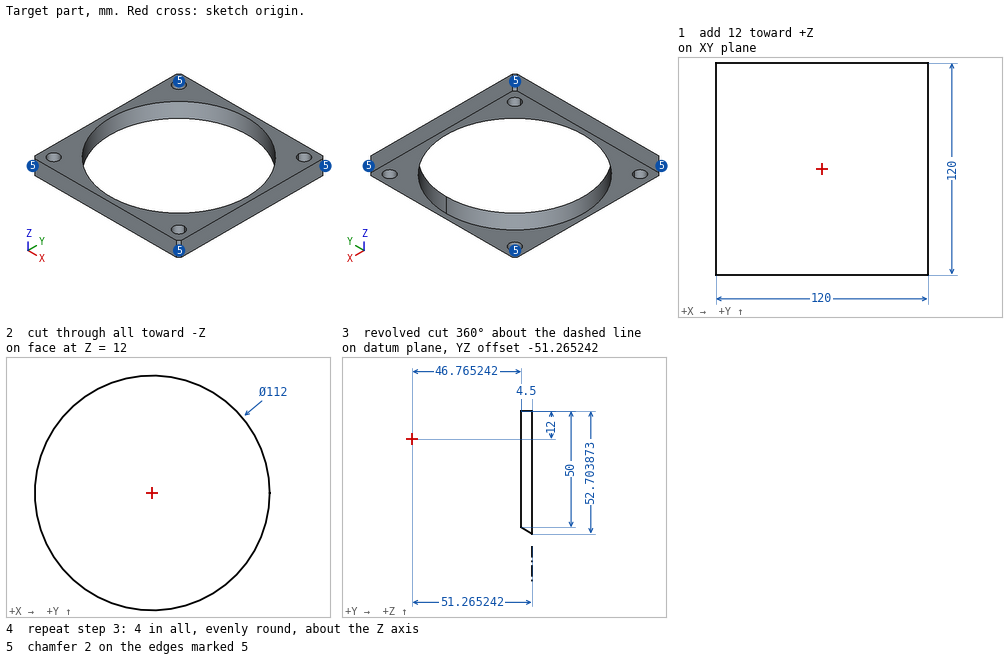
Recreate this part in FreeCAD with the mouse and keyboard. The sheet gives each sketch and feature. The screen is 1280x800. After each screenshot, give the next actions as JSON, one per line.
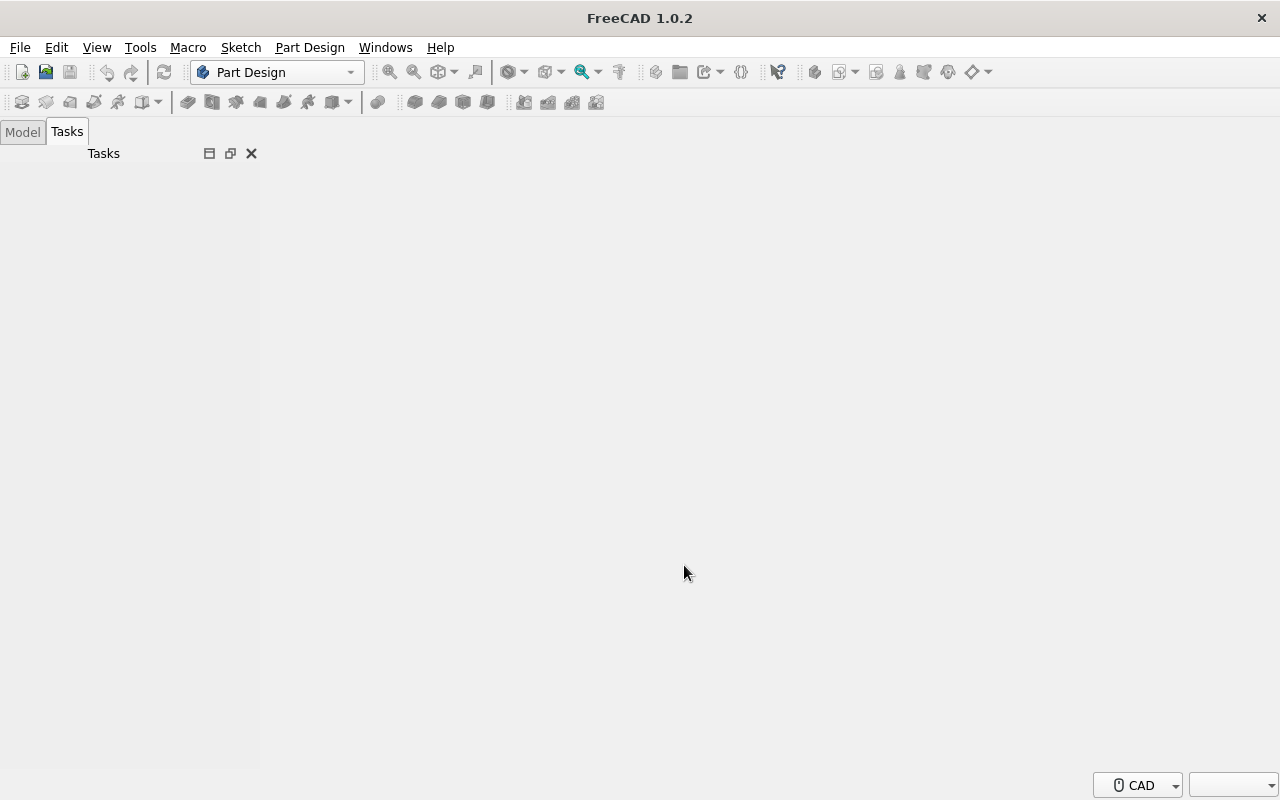
{"action": "key", "text": "ctrl+n"}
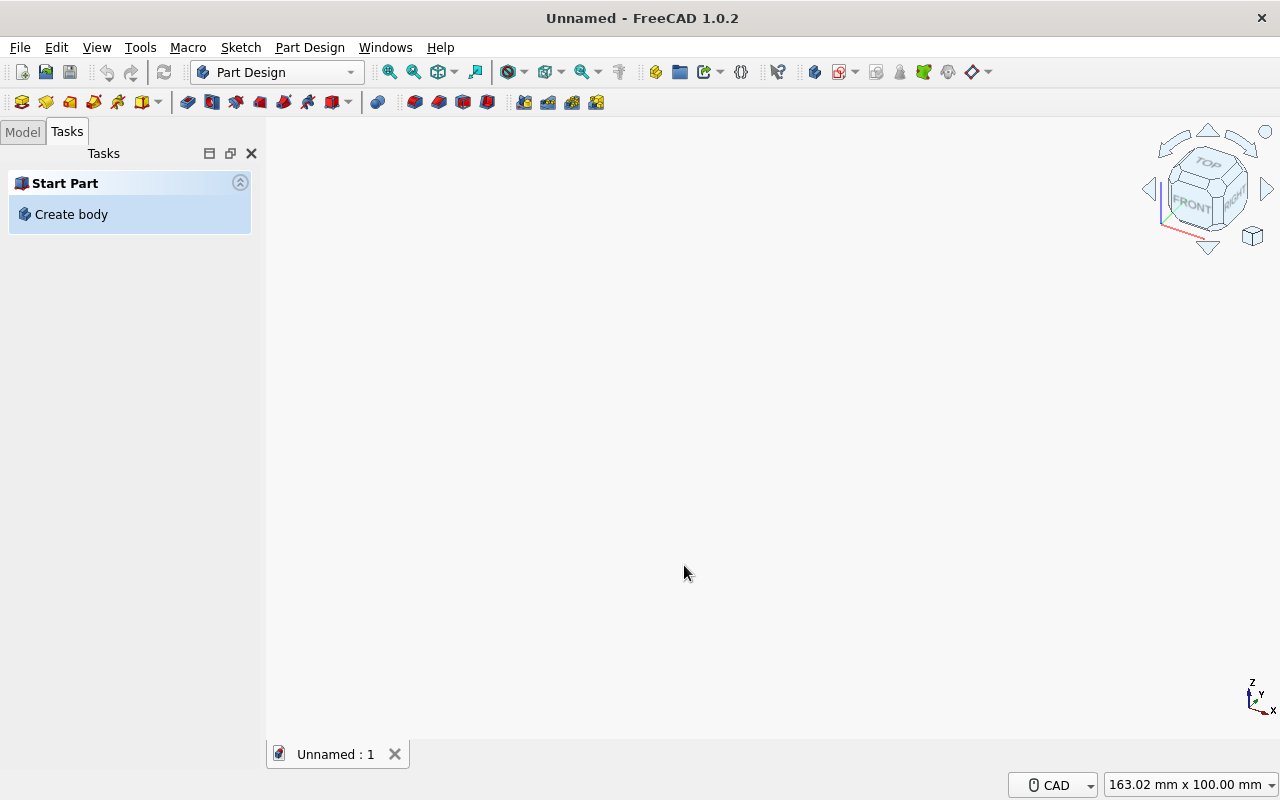
{"action": "left_click", "coordinate": [840, 72]}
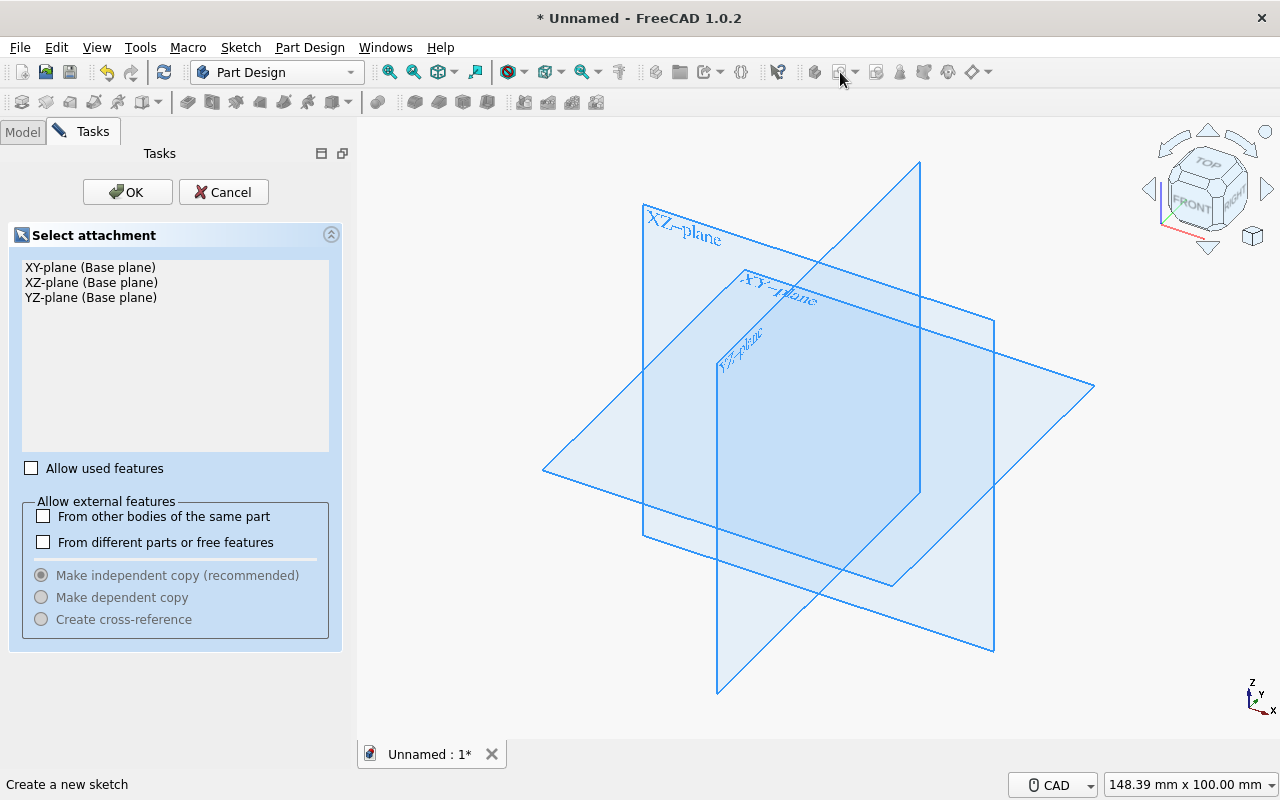
{"action": "left_click", "coordinate": [82, 268]}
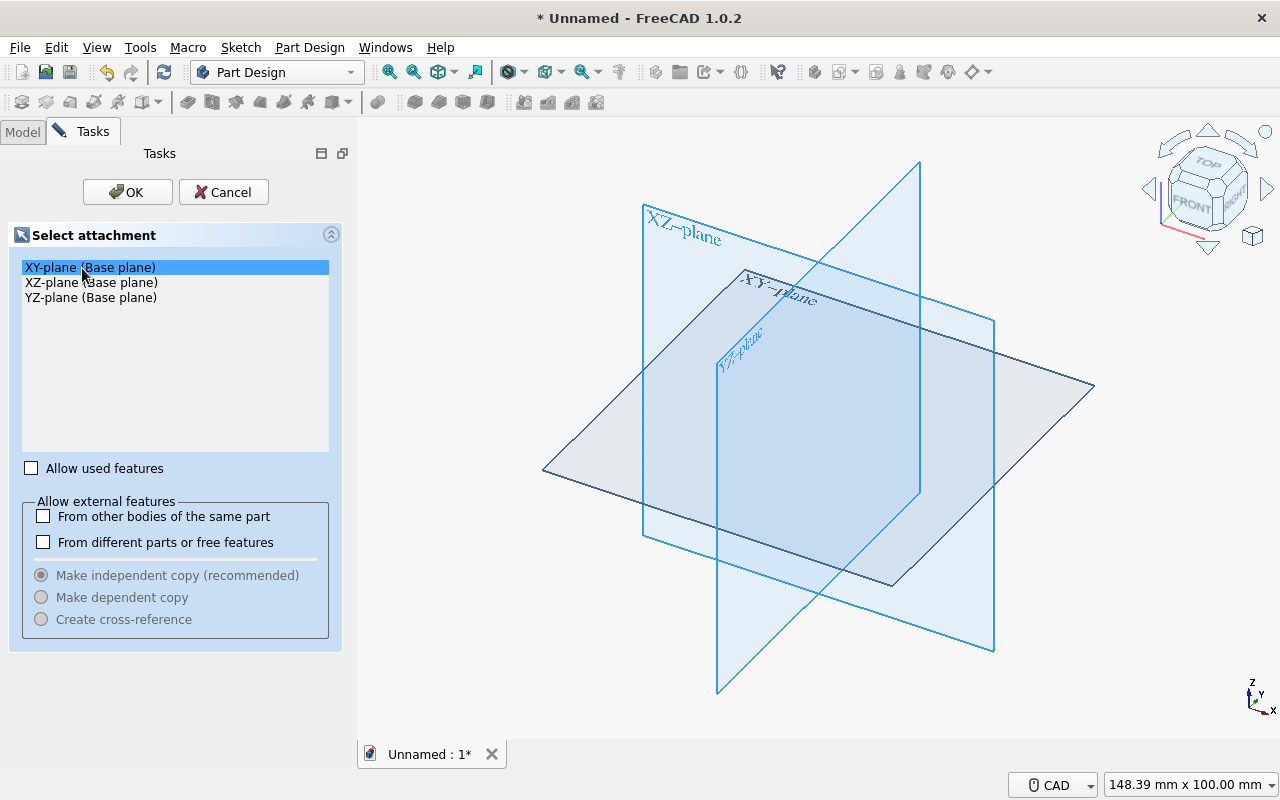
{"action": "left_click", "coordinate": [128, 192]}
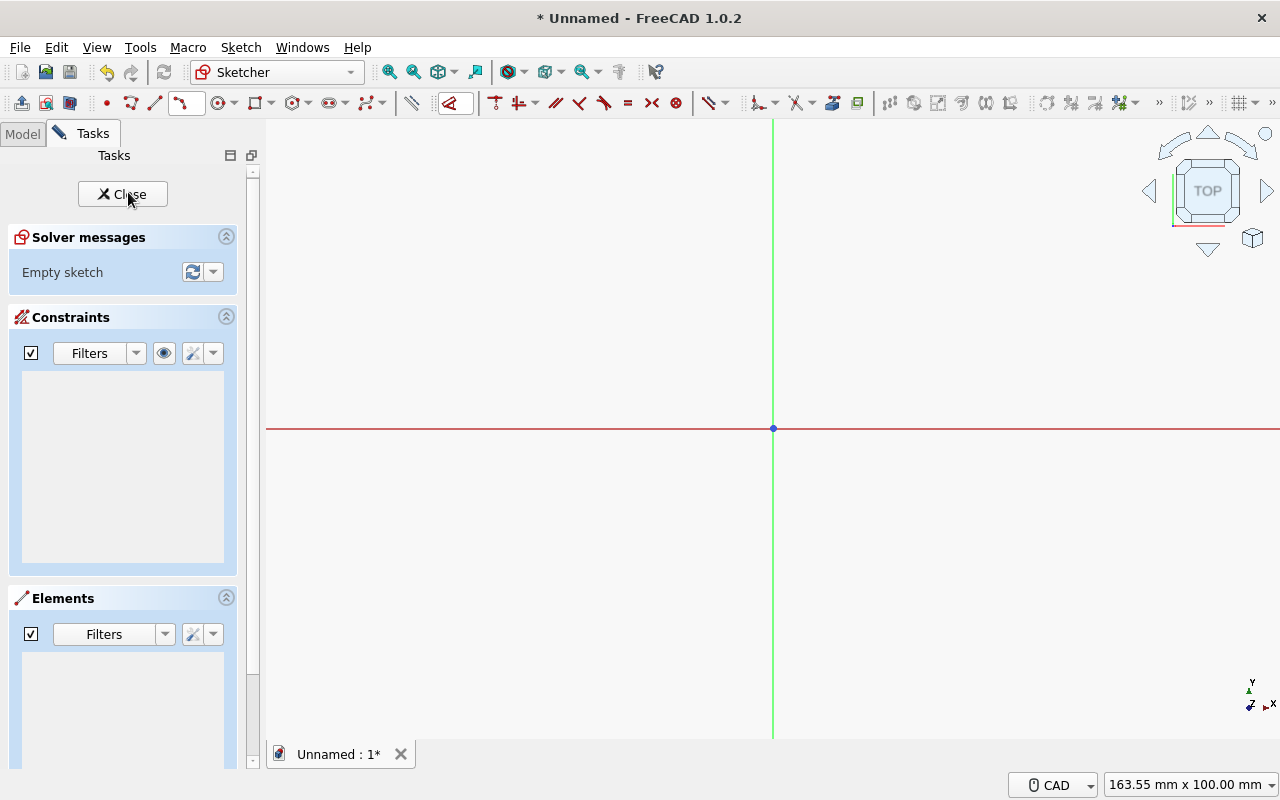
{"action": "scroll", "coordinate": [621, 429], "scroll_direction": "down", "scroll_amount": 3}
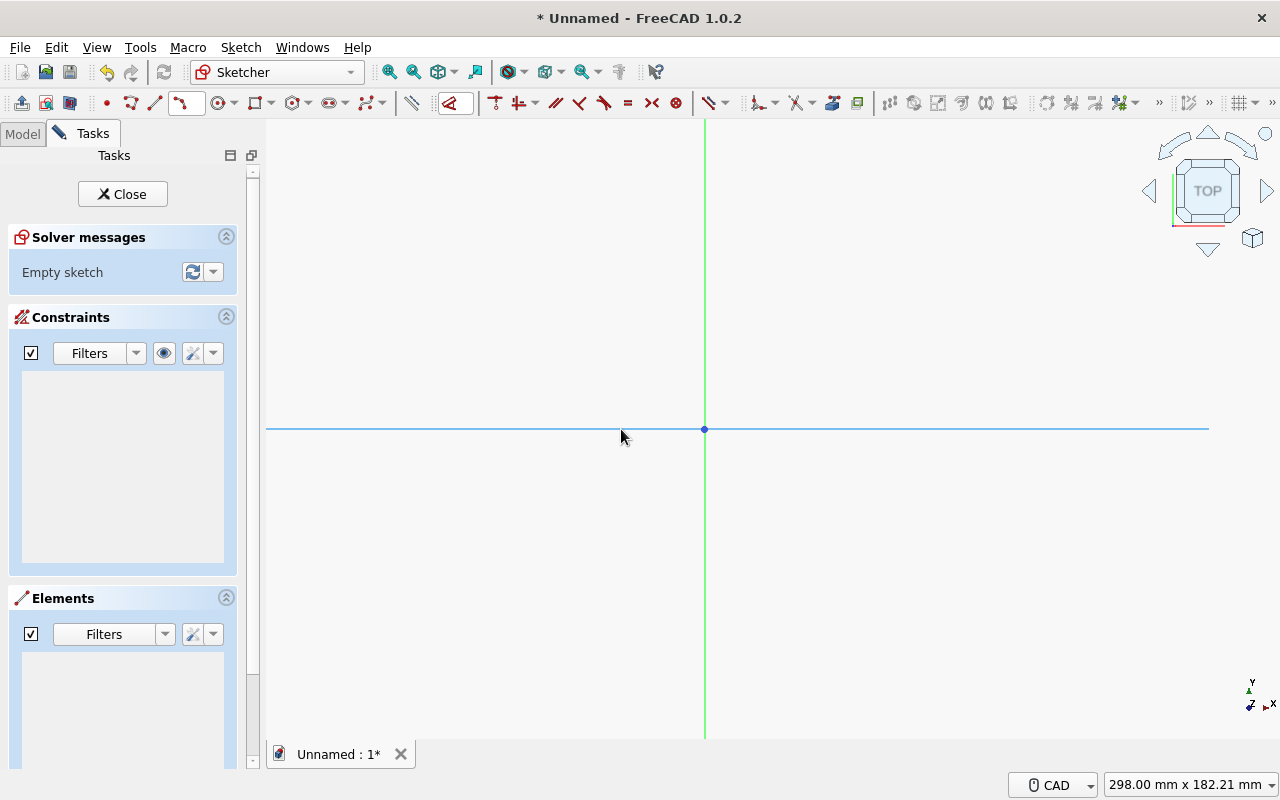
{"action": "left_click", "coordinate": [274, 104]}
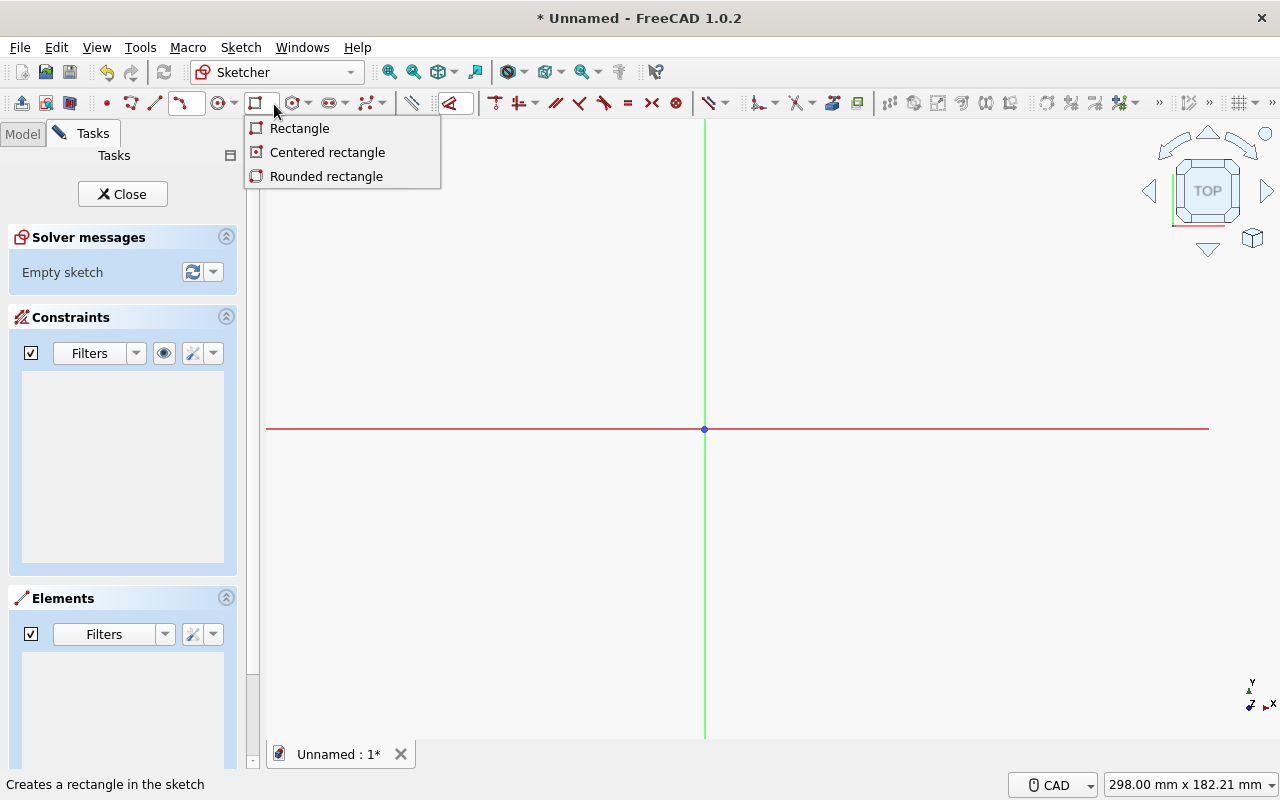
{"action": "left_click", "coordinate": [342, 152]}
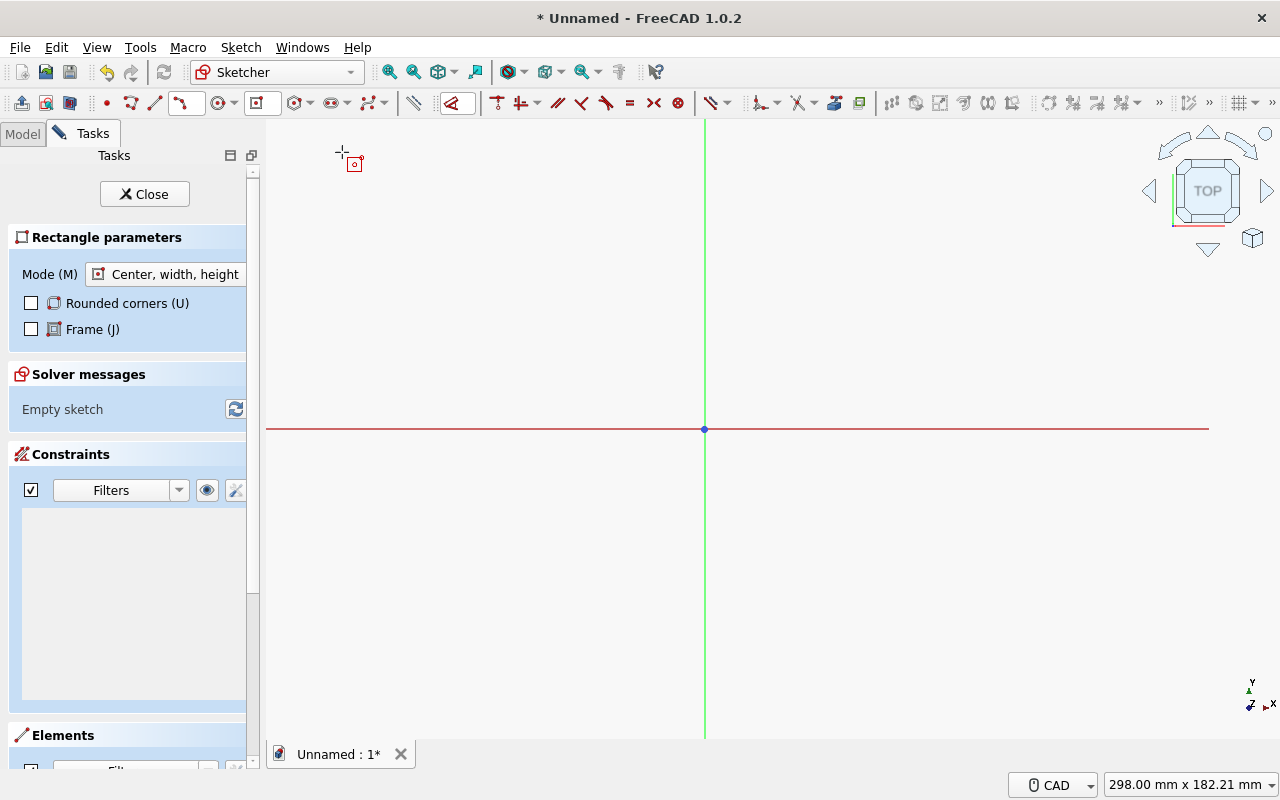
{"action": "left_click", "coordinate": [705, 429]}
{"action": "mouse_move", "coordinate": [909, 225]}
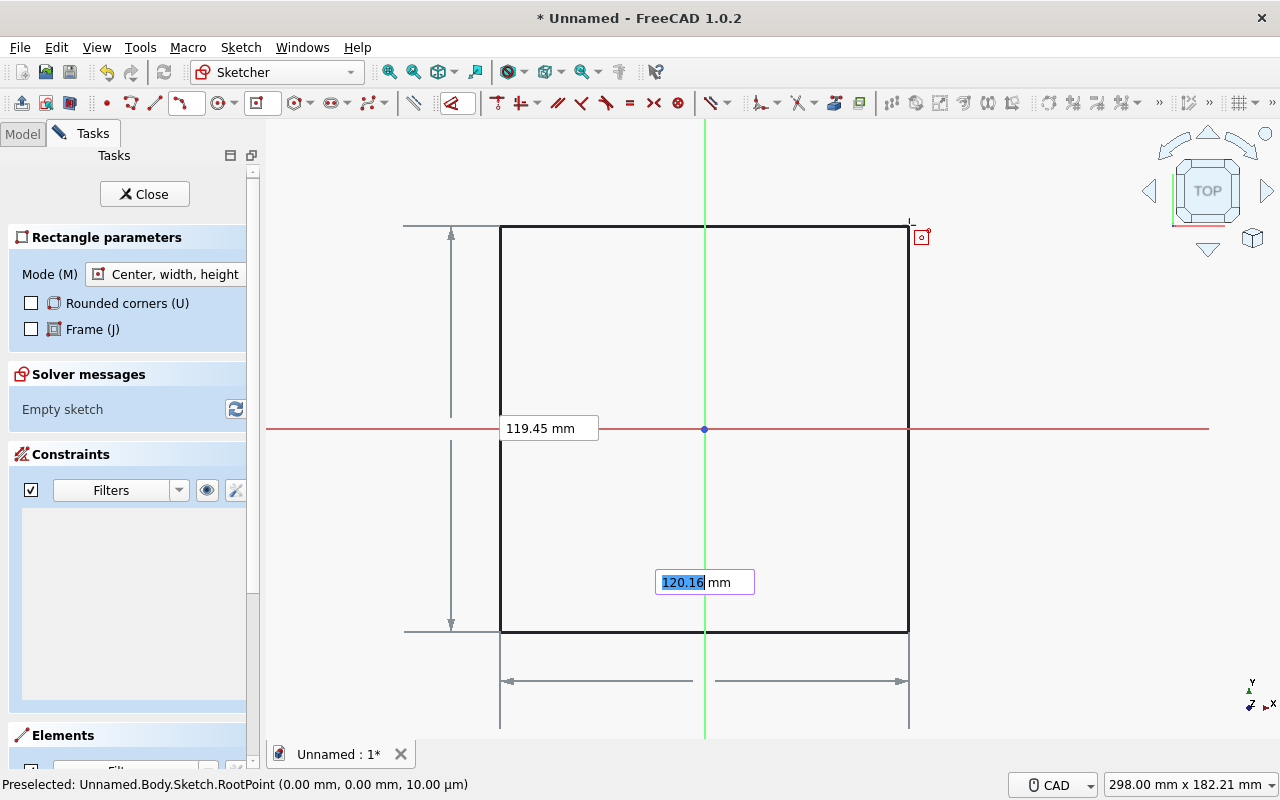
{"action": "type", "text": "120"}
{"action": "key", "text": "Tab"}
{"action": "type", "text": "120"}
{"action": "key", "text": "Return"}
{"action": "key", "text": "Escape"}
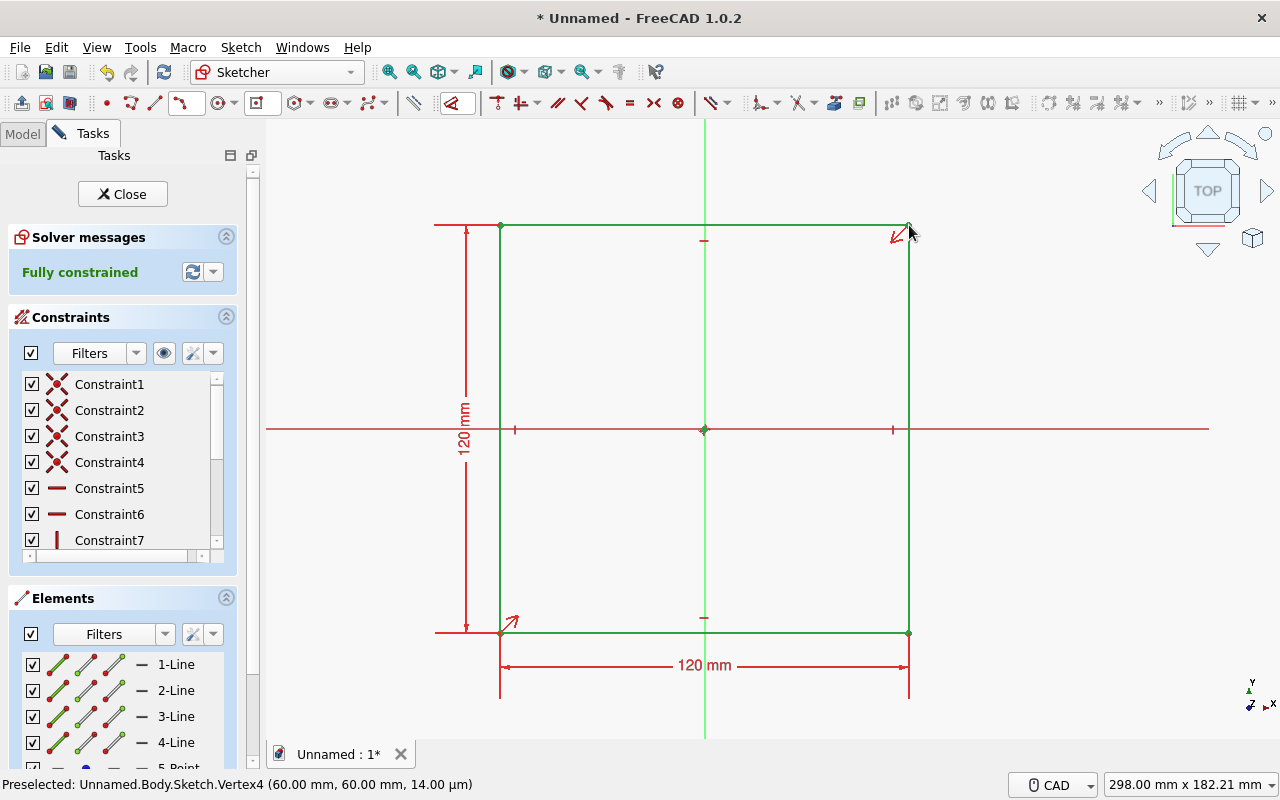
{"action": "left_click", "coordinate": [123, 194]}